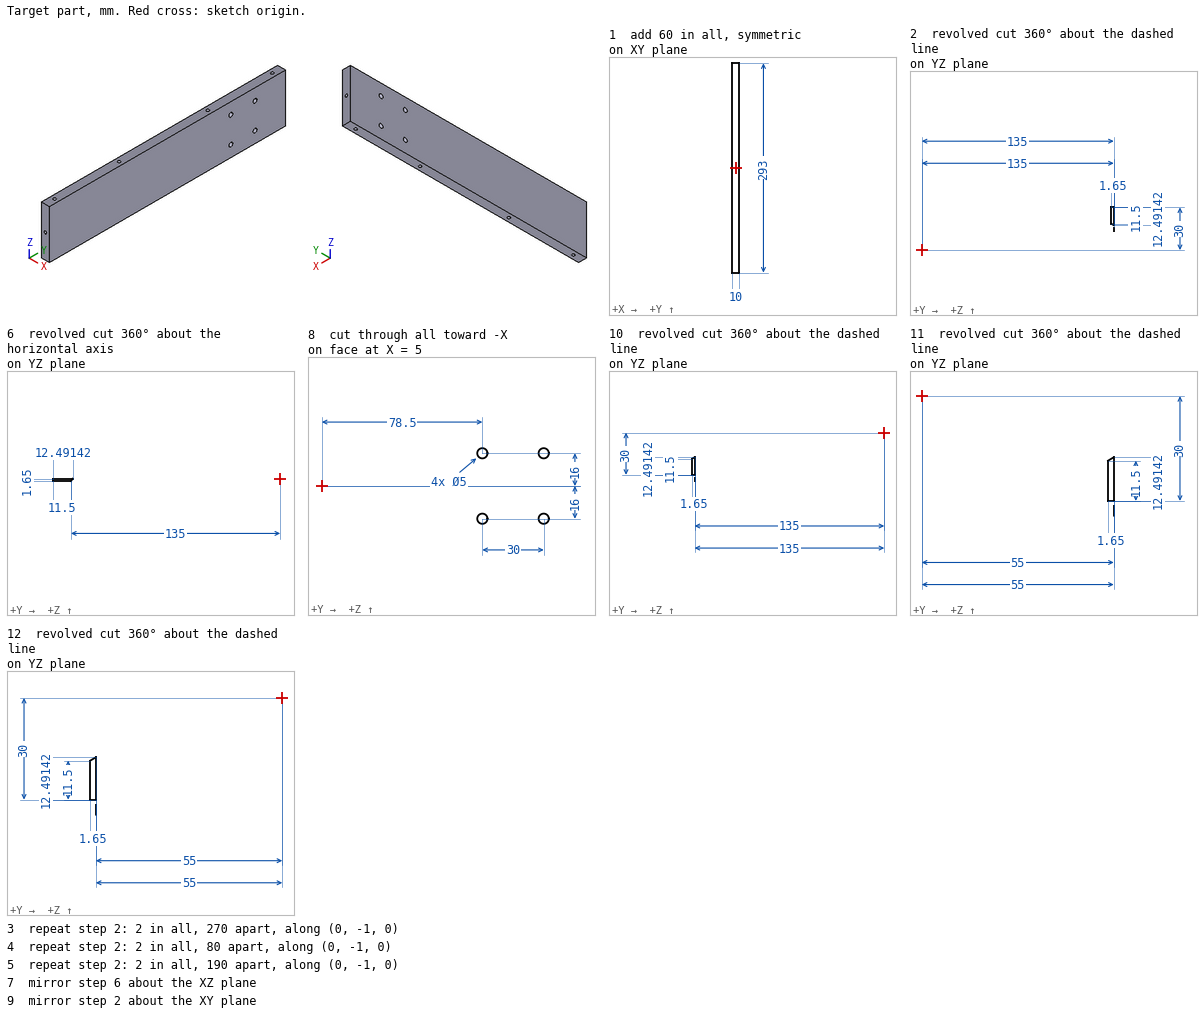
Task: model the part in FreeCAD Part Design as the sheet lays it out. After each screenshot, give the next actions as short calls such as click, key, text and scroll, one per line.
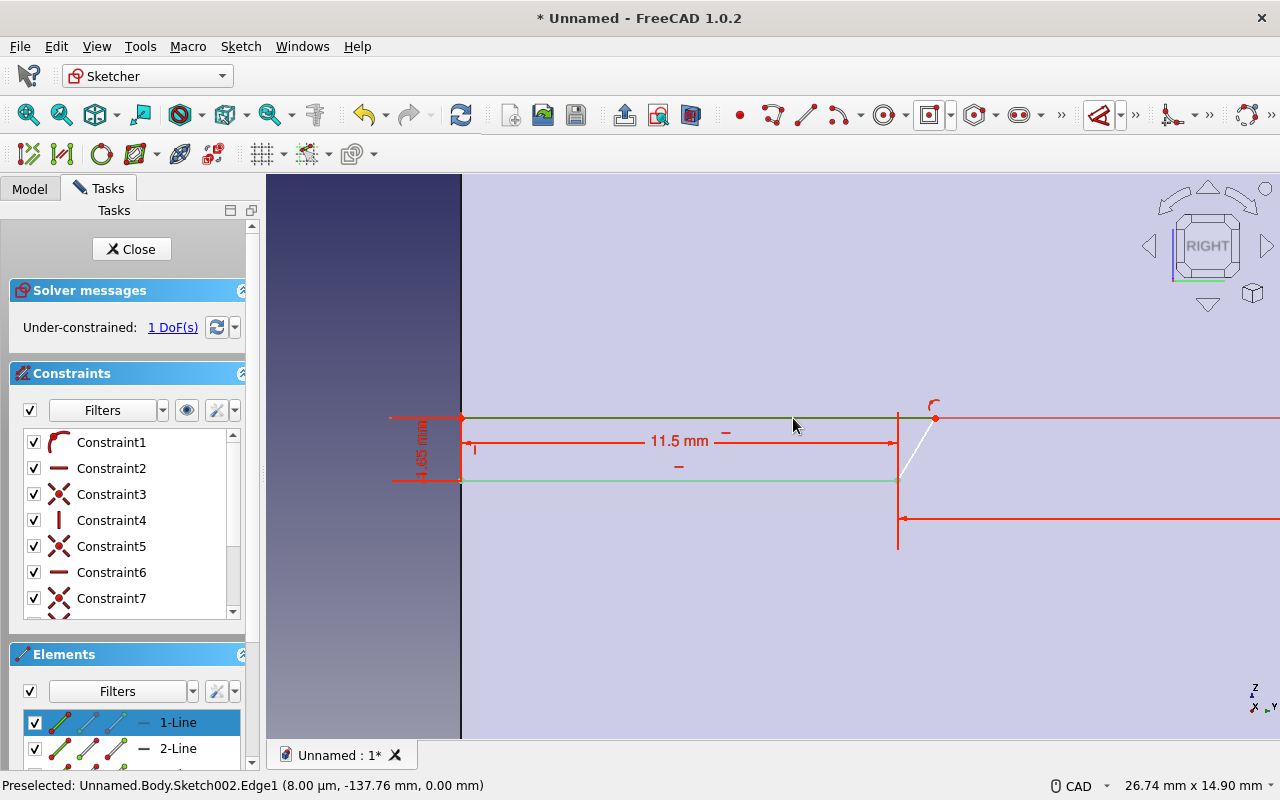
click(1120, 116)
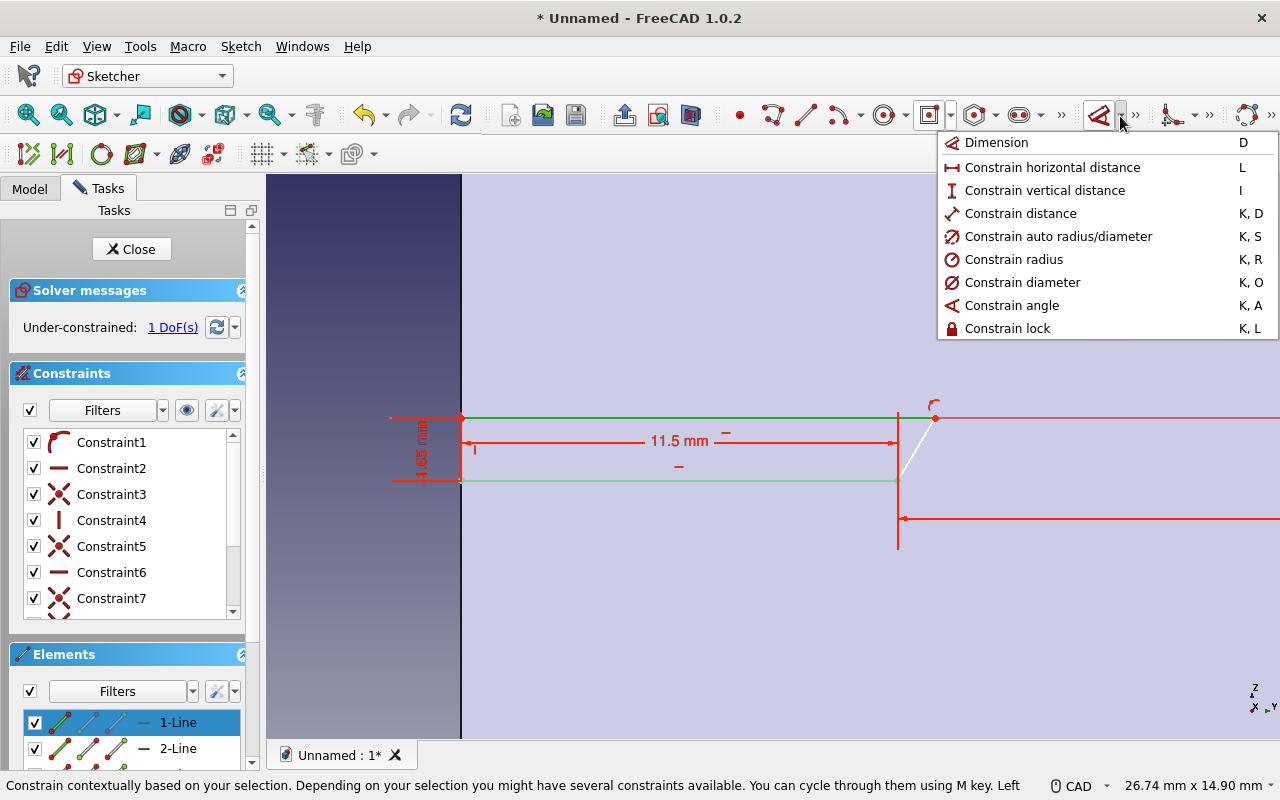
click(1108, 168)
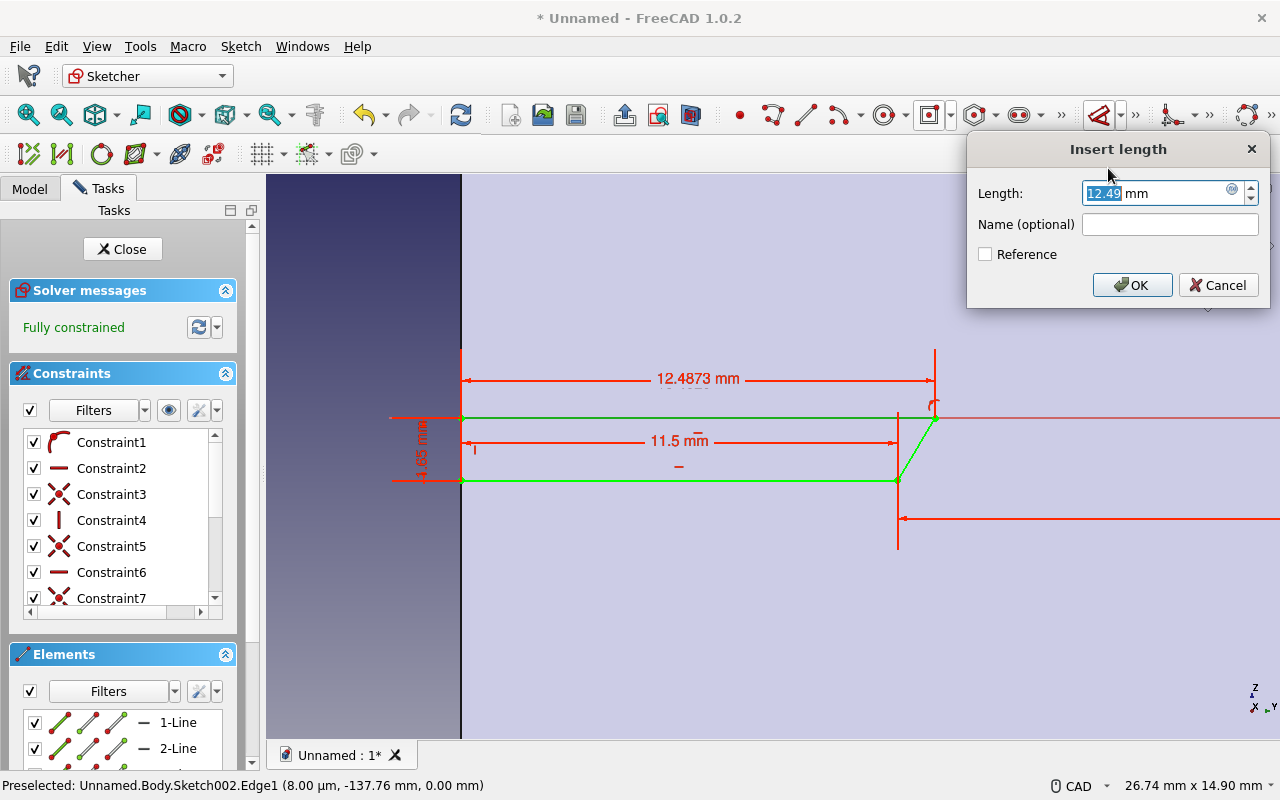
text(12.49142)
key(Return)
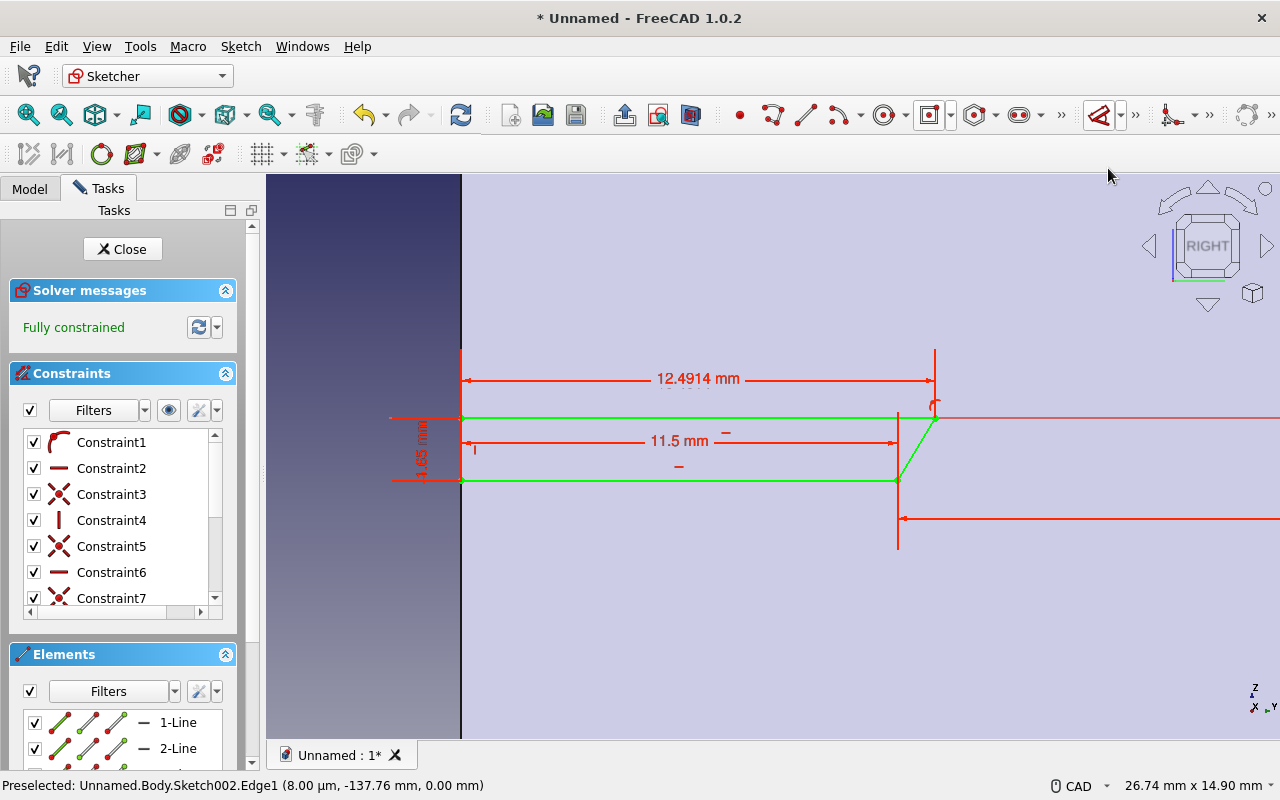
click(123, 249)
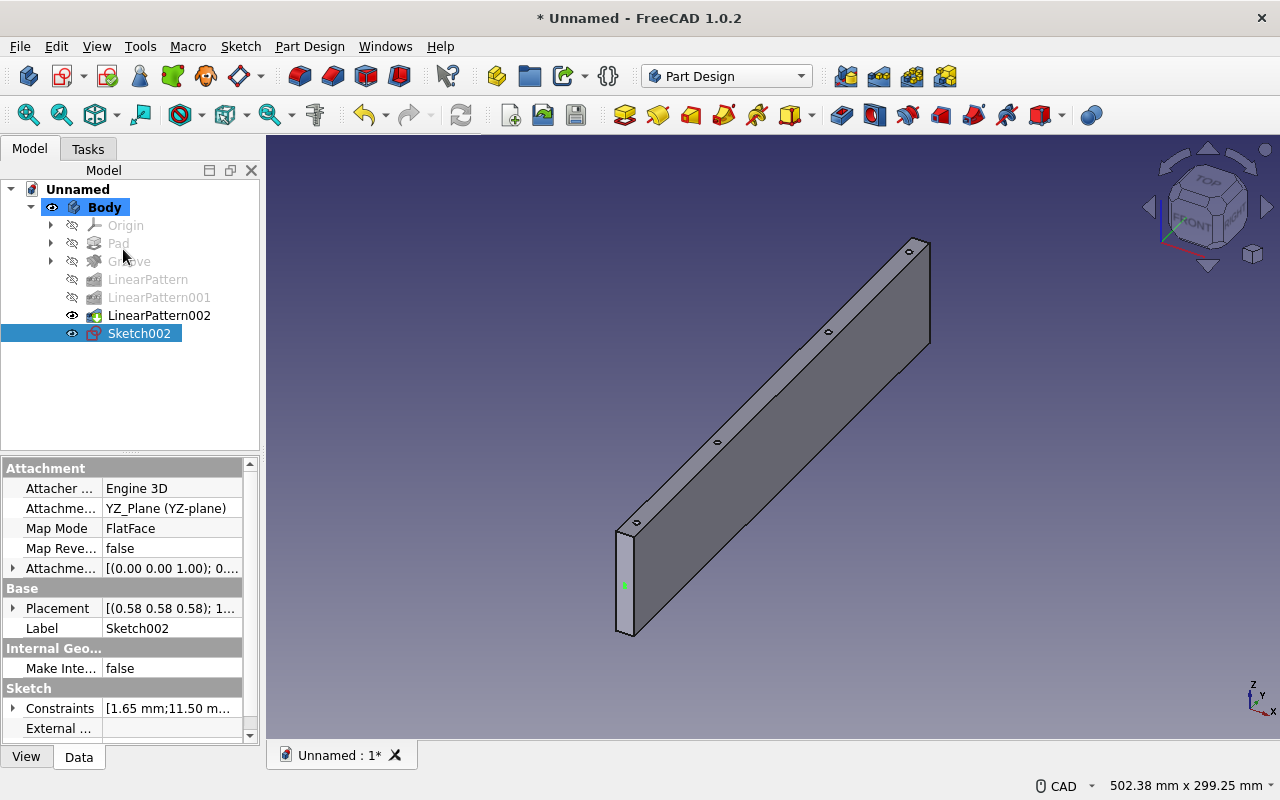
click(908, 116)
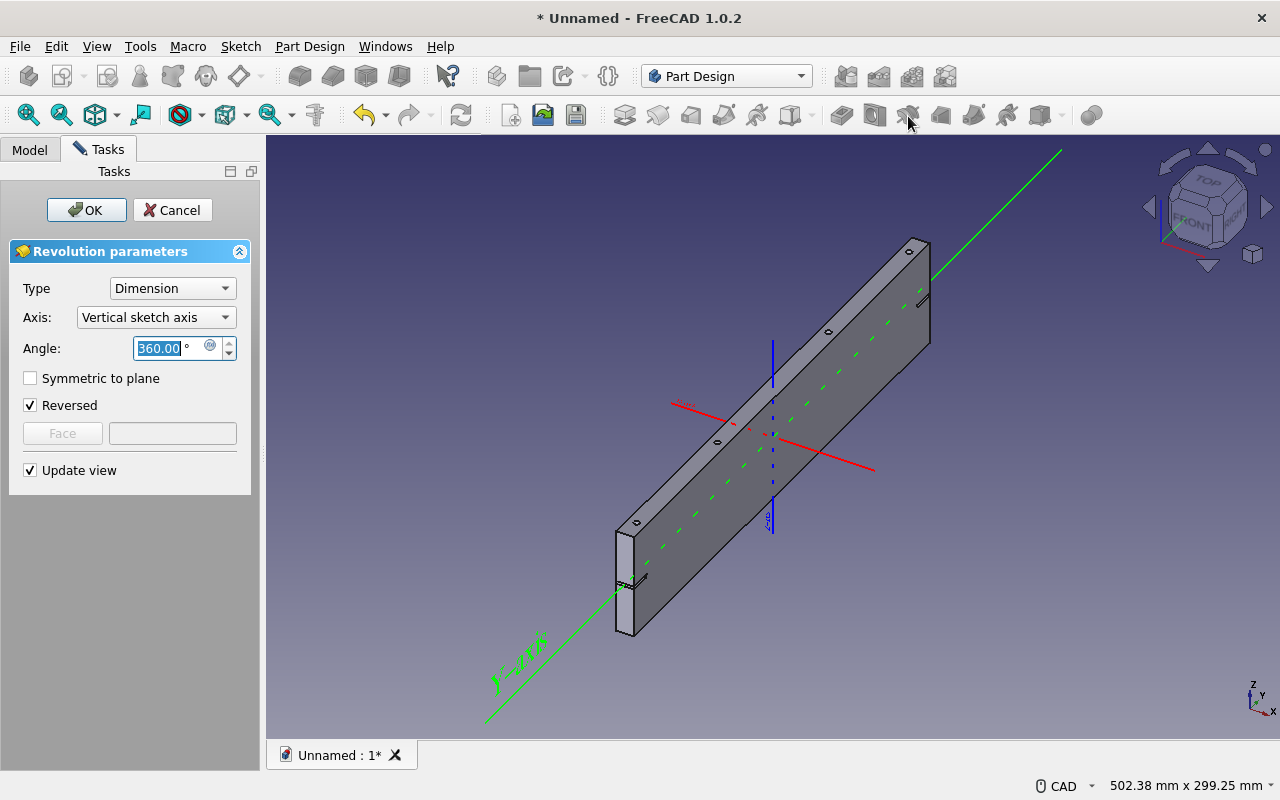
click(157, 318)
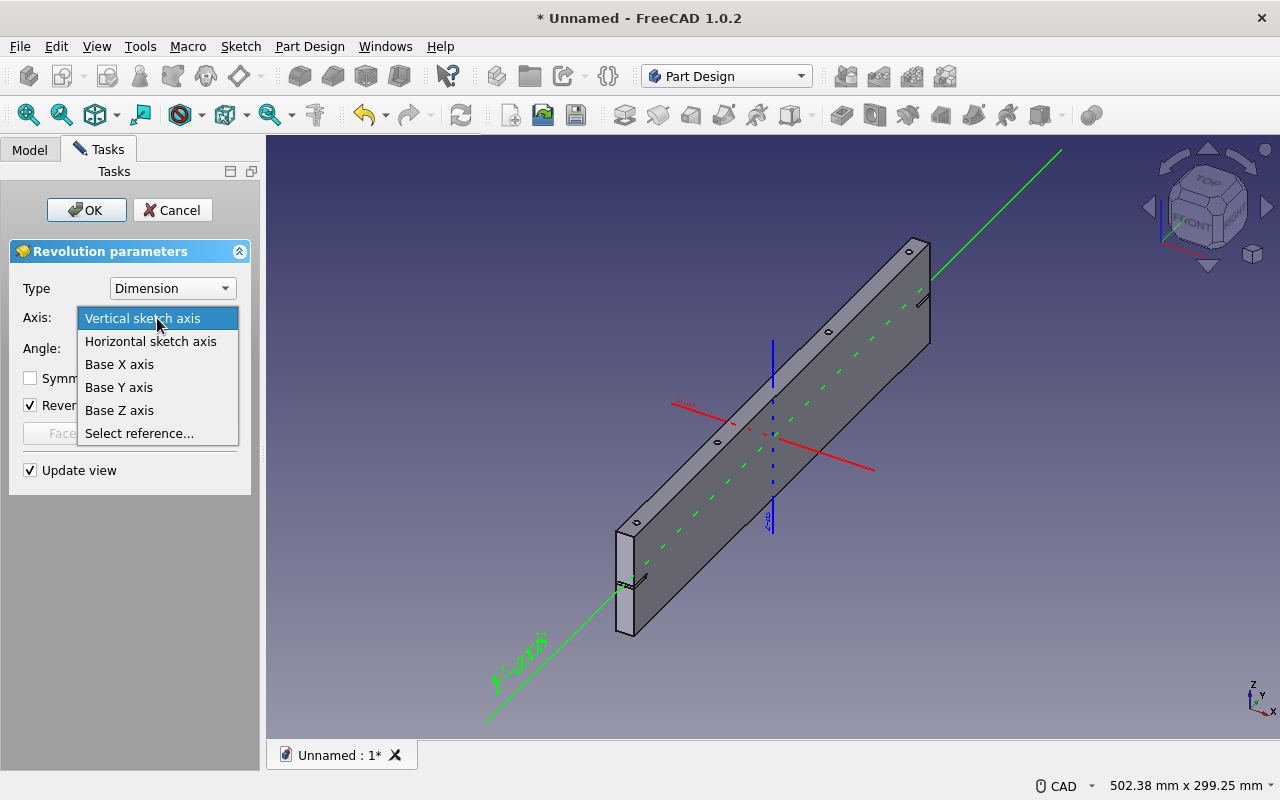
click(156, 342)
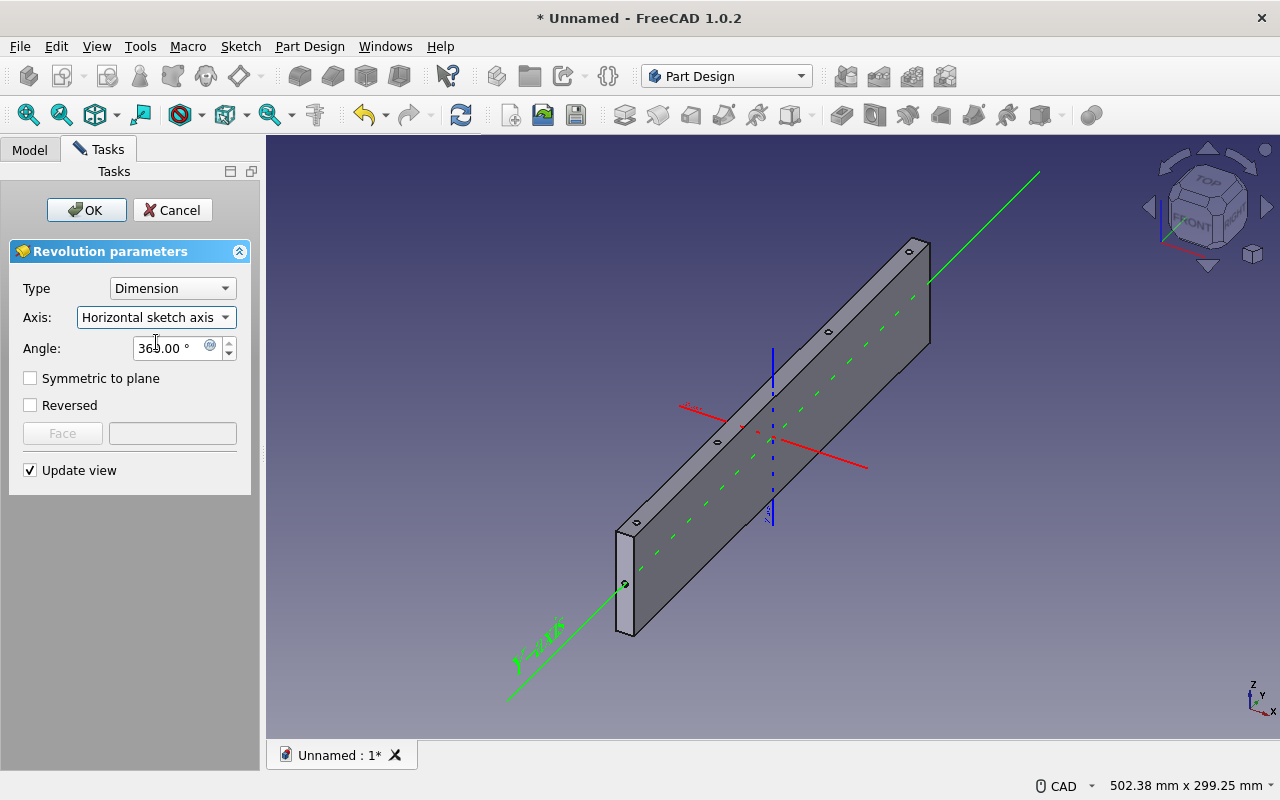
click(87, 210)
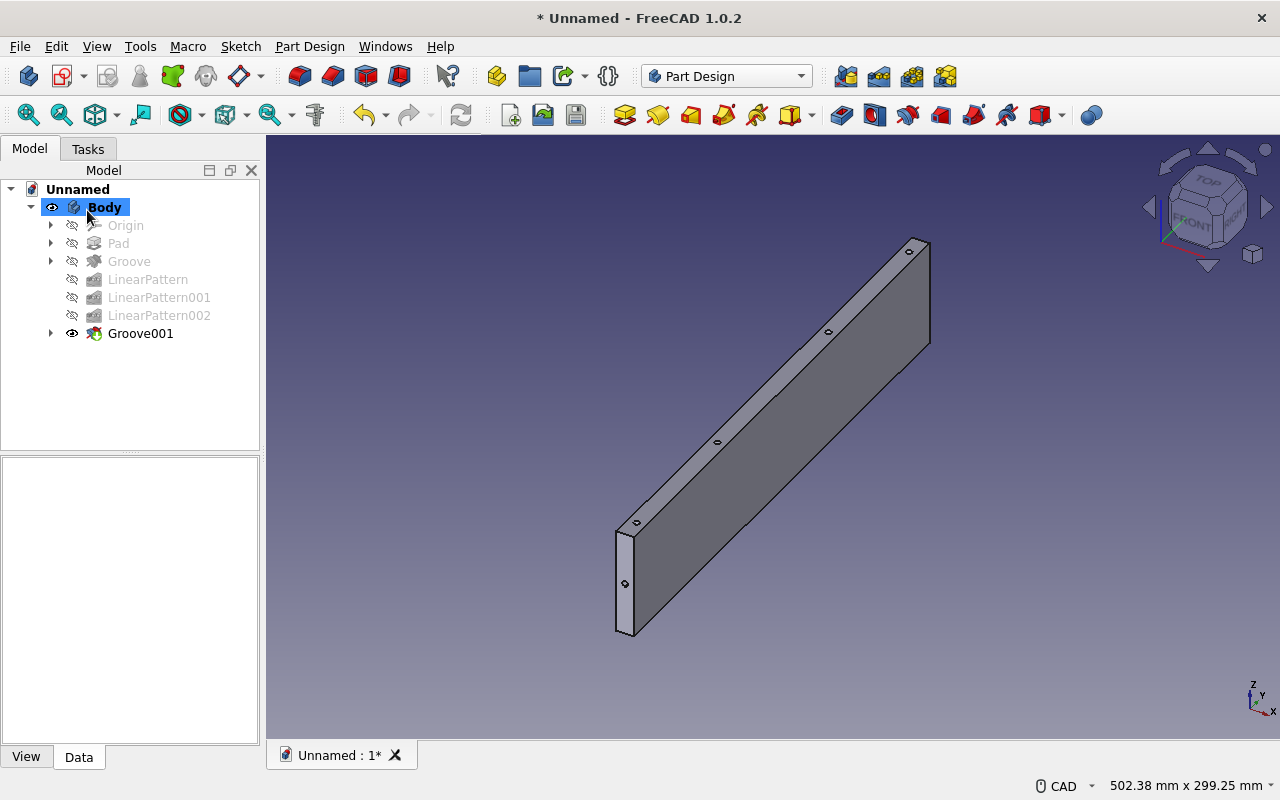
click(117, 333)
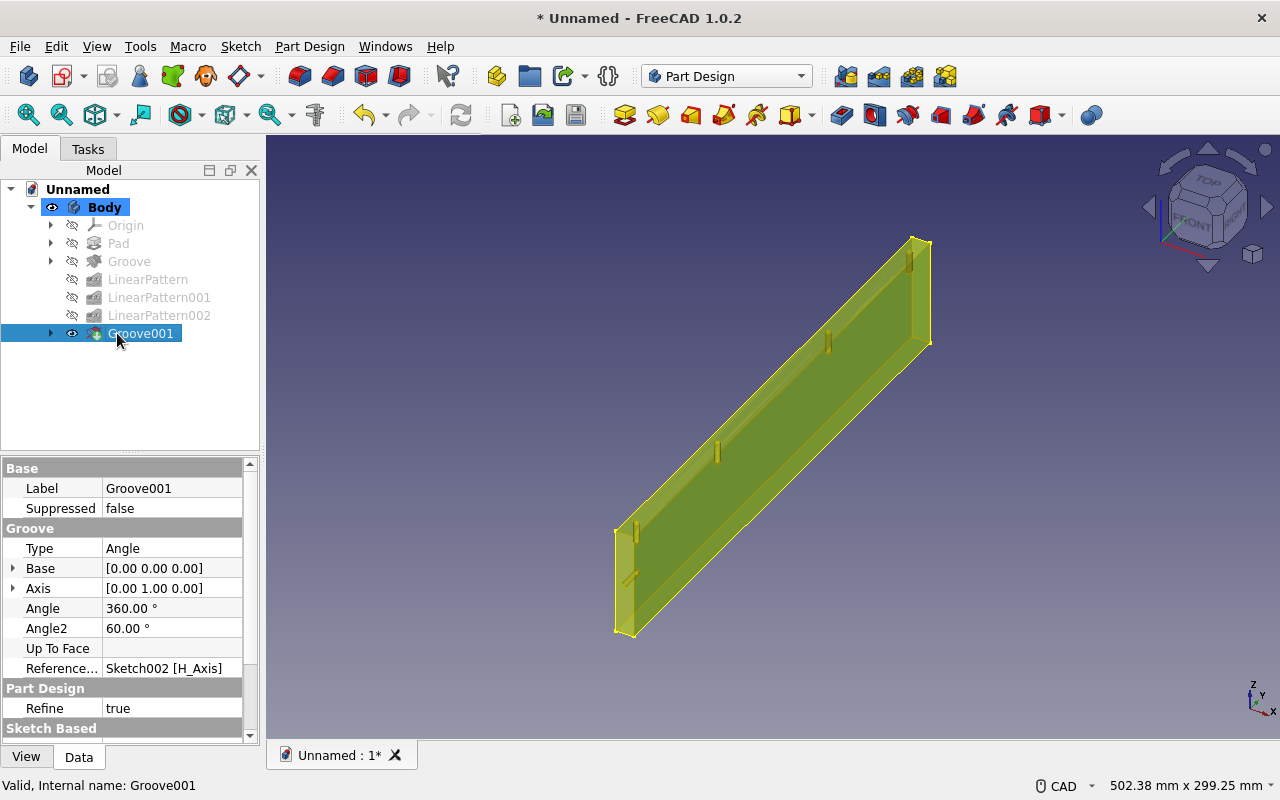
click(846, 76)